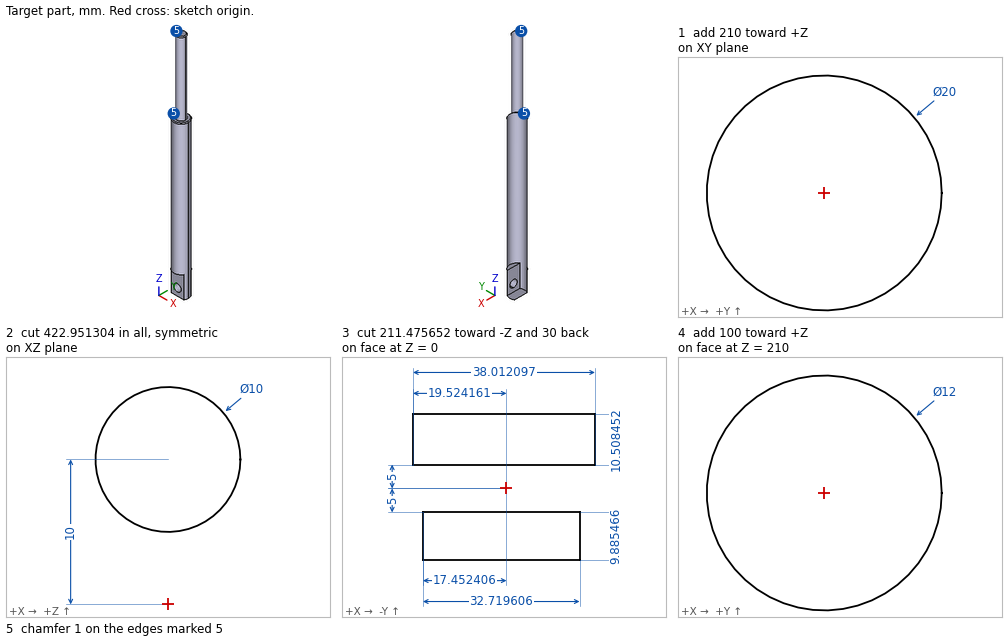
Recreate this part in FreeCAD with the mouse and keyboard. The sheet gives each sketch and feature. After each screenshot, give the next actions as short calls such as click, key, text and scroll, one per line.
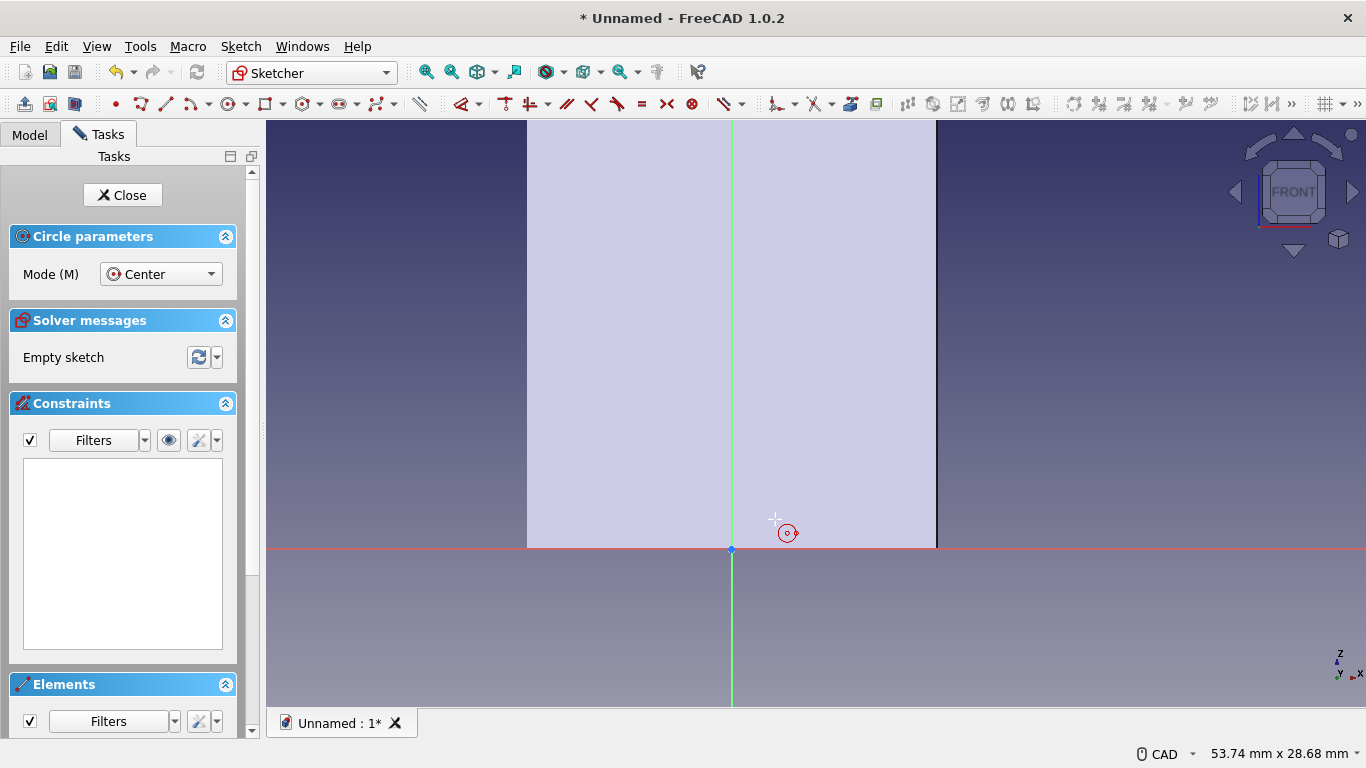
click(732, 344)
move(804, 272)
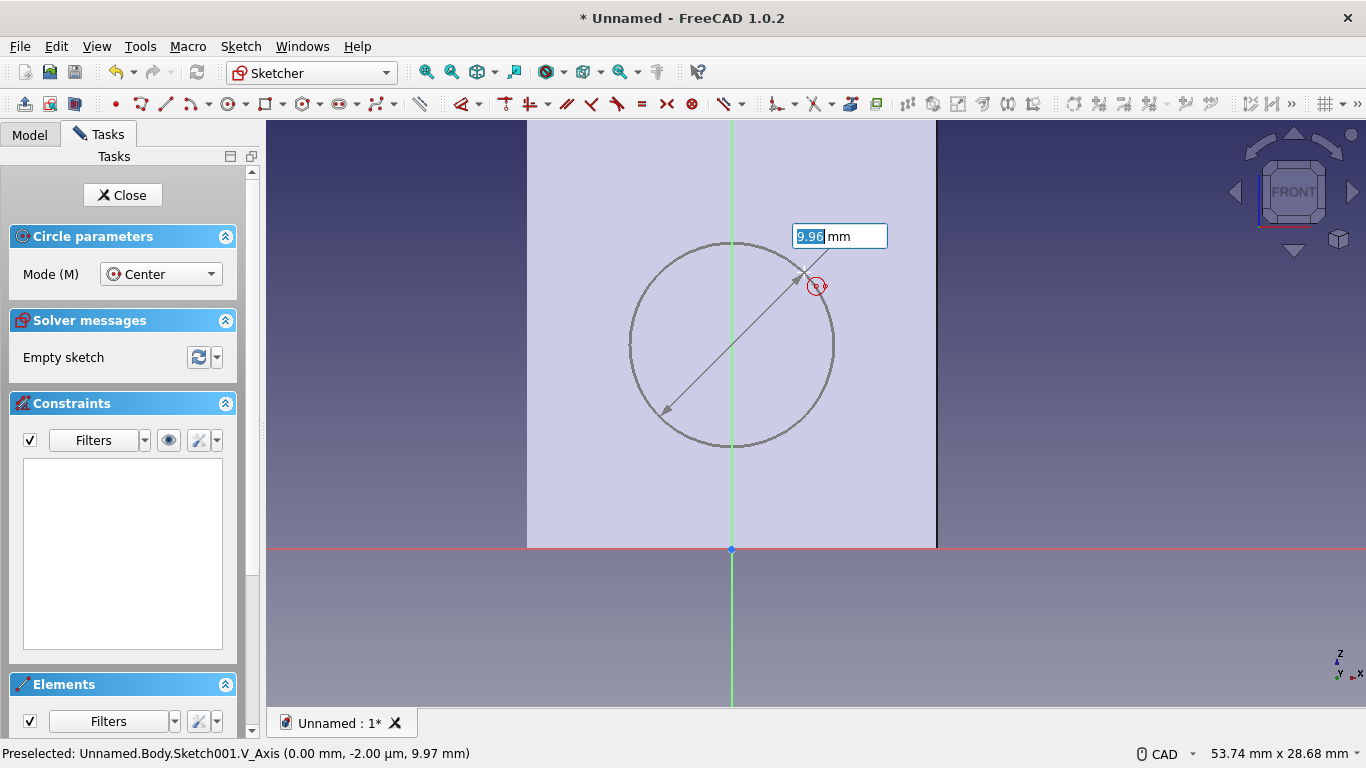
text(10)
key(Return)
key(Escape)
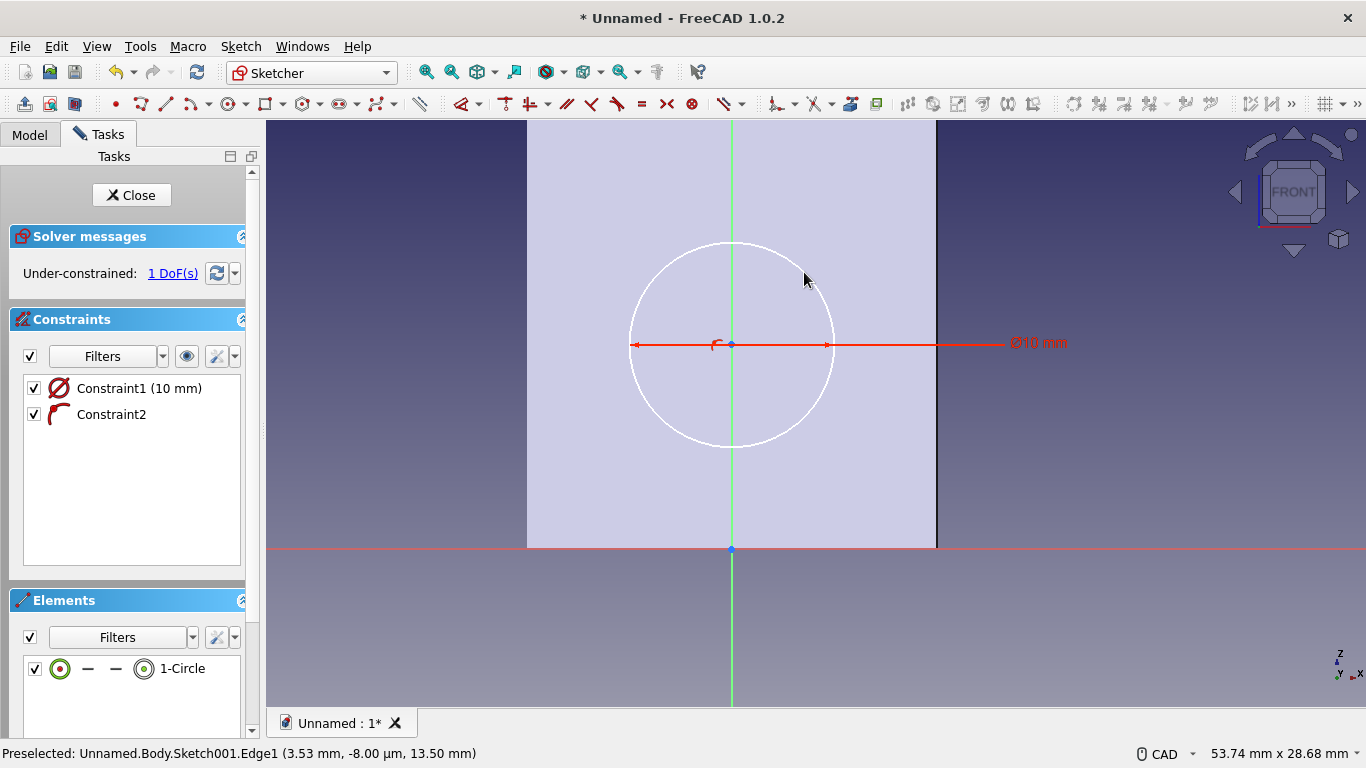
click(732, 345)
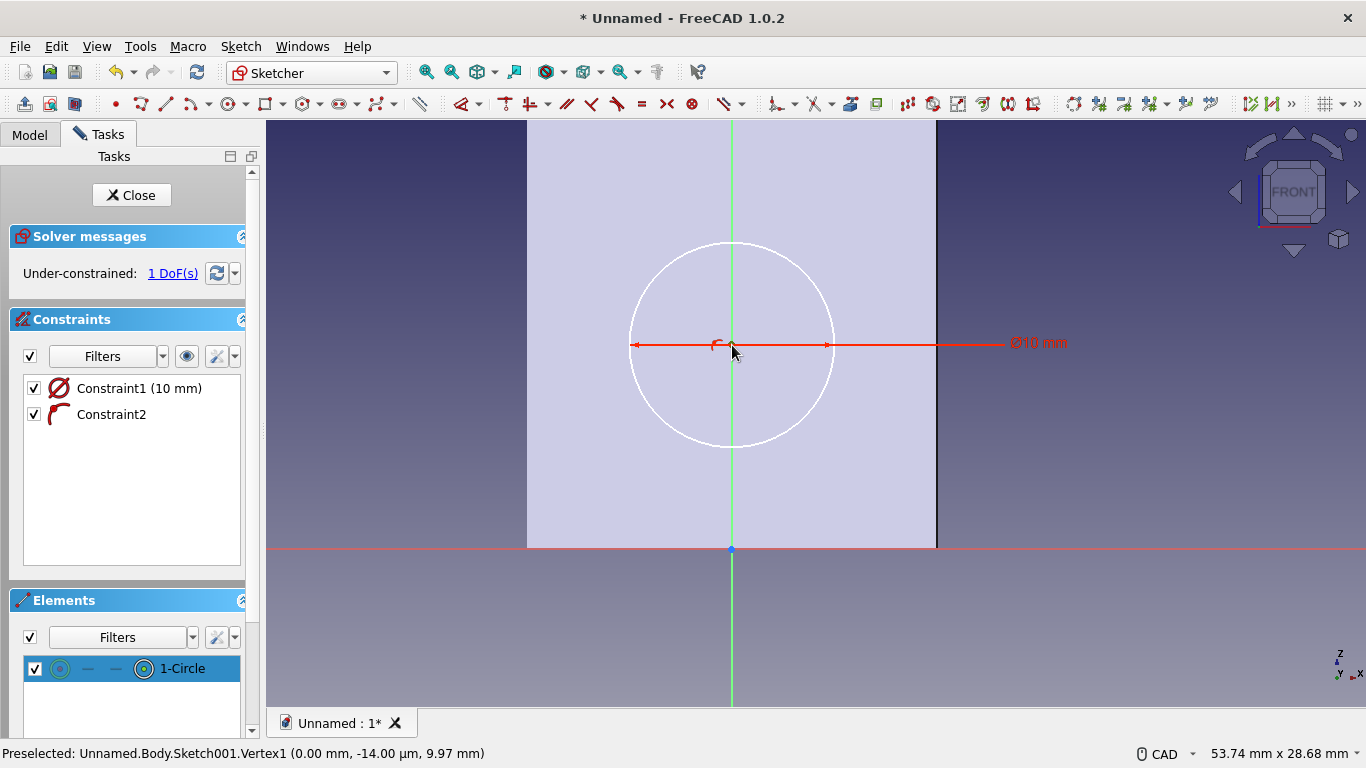
click(478, 104)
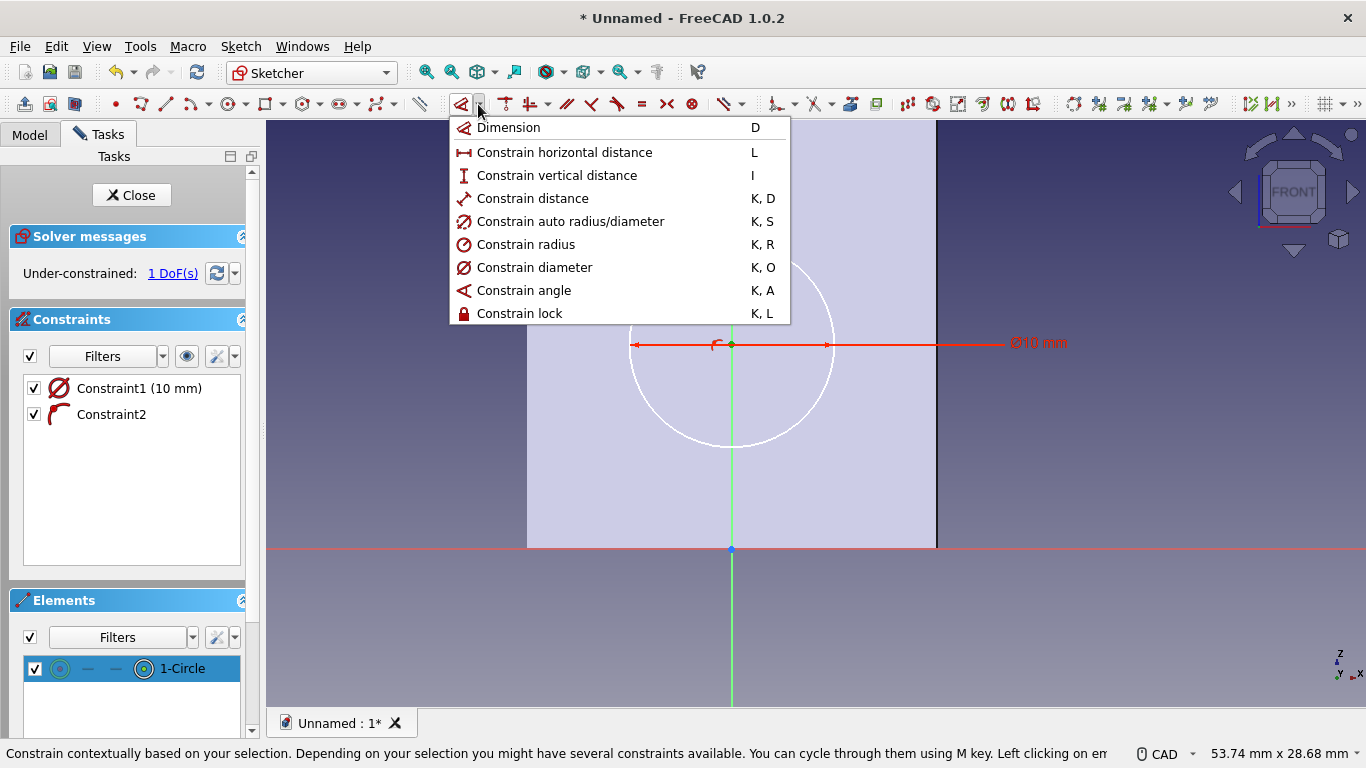
click(620, 176)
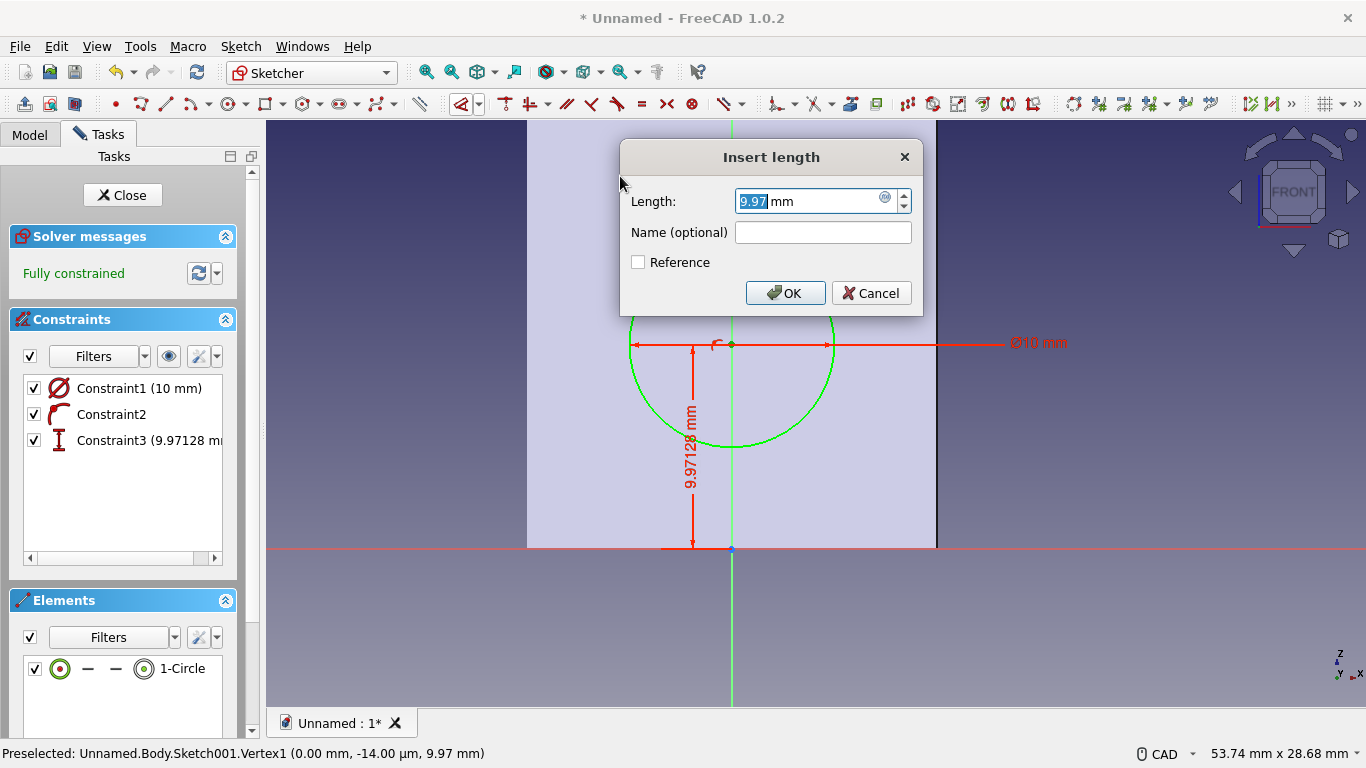
text(10)
key(Return)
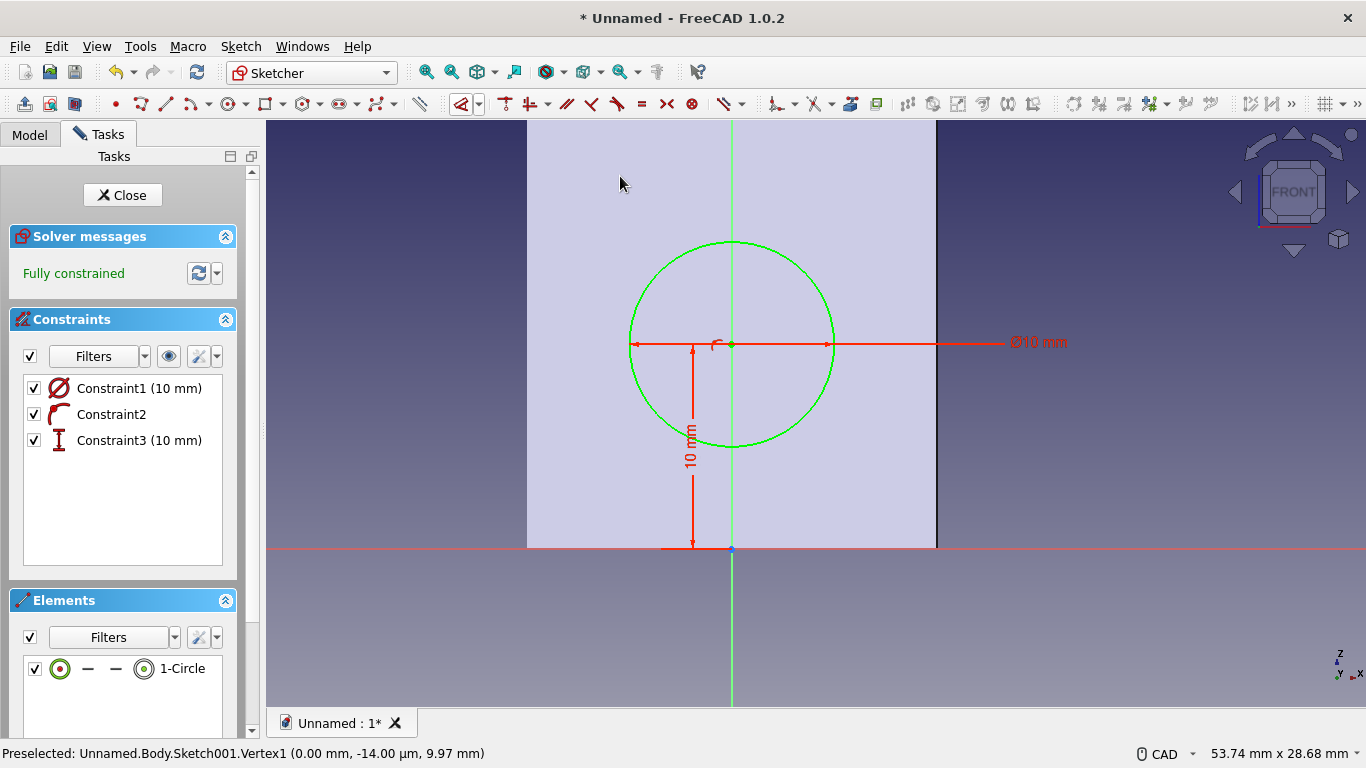
click(123, 195)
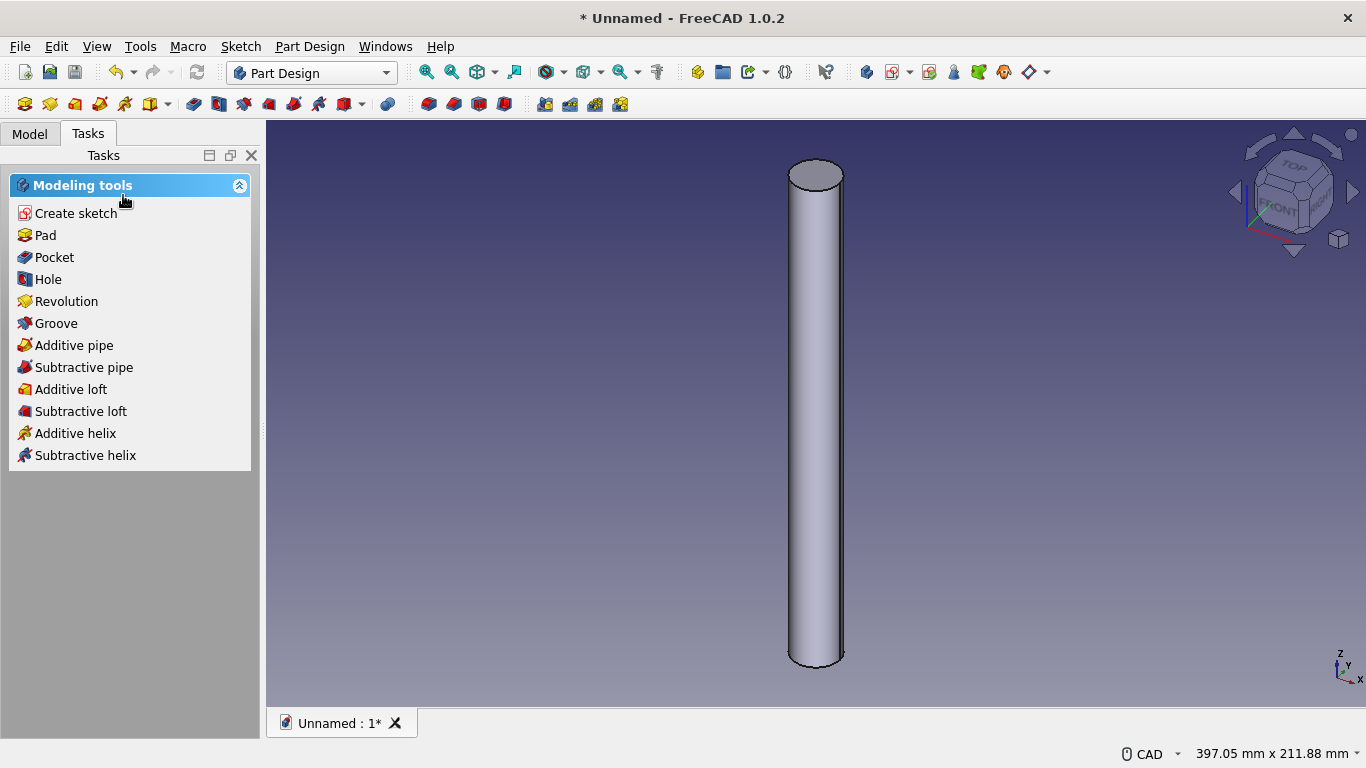
click(194, 104)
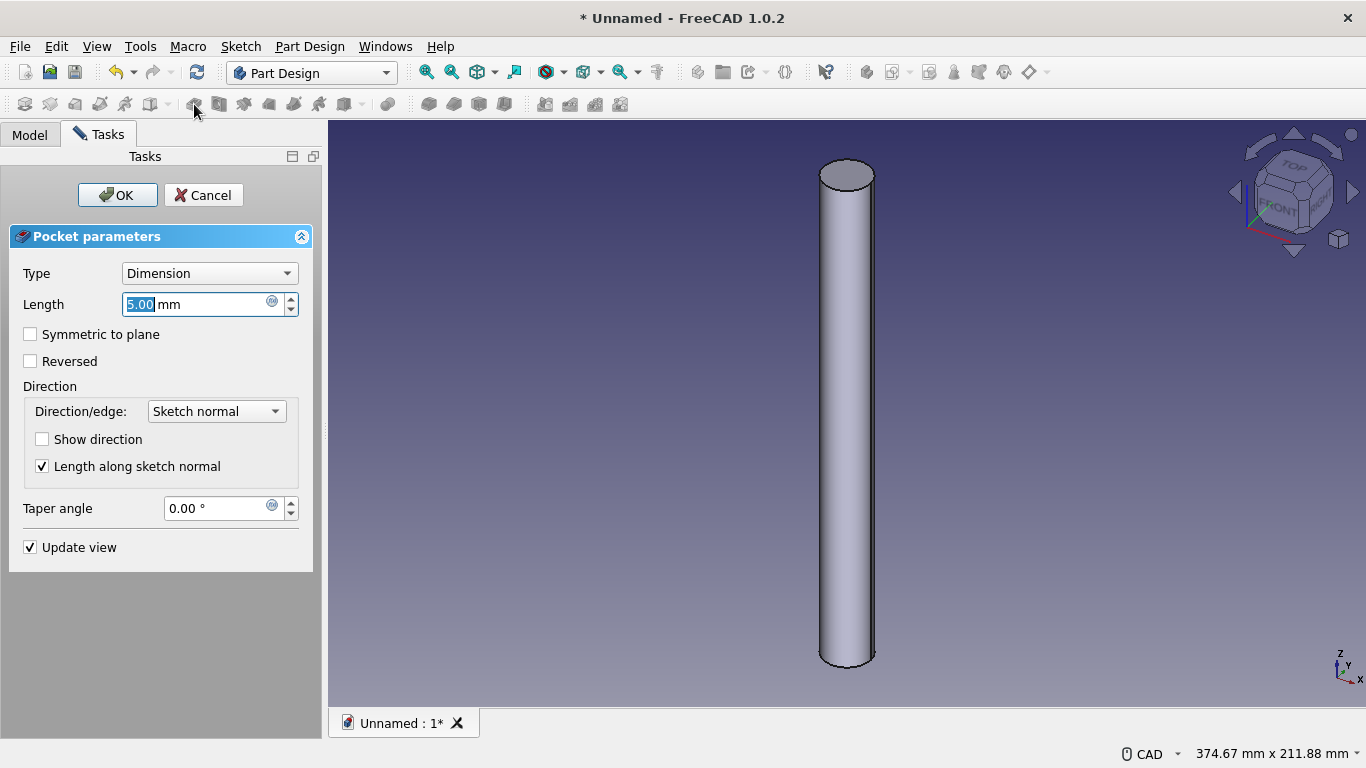
text(422.951304)
key(Tab)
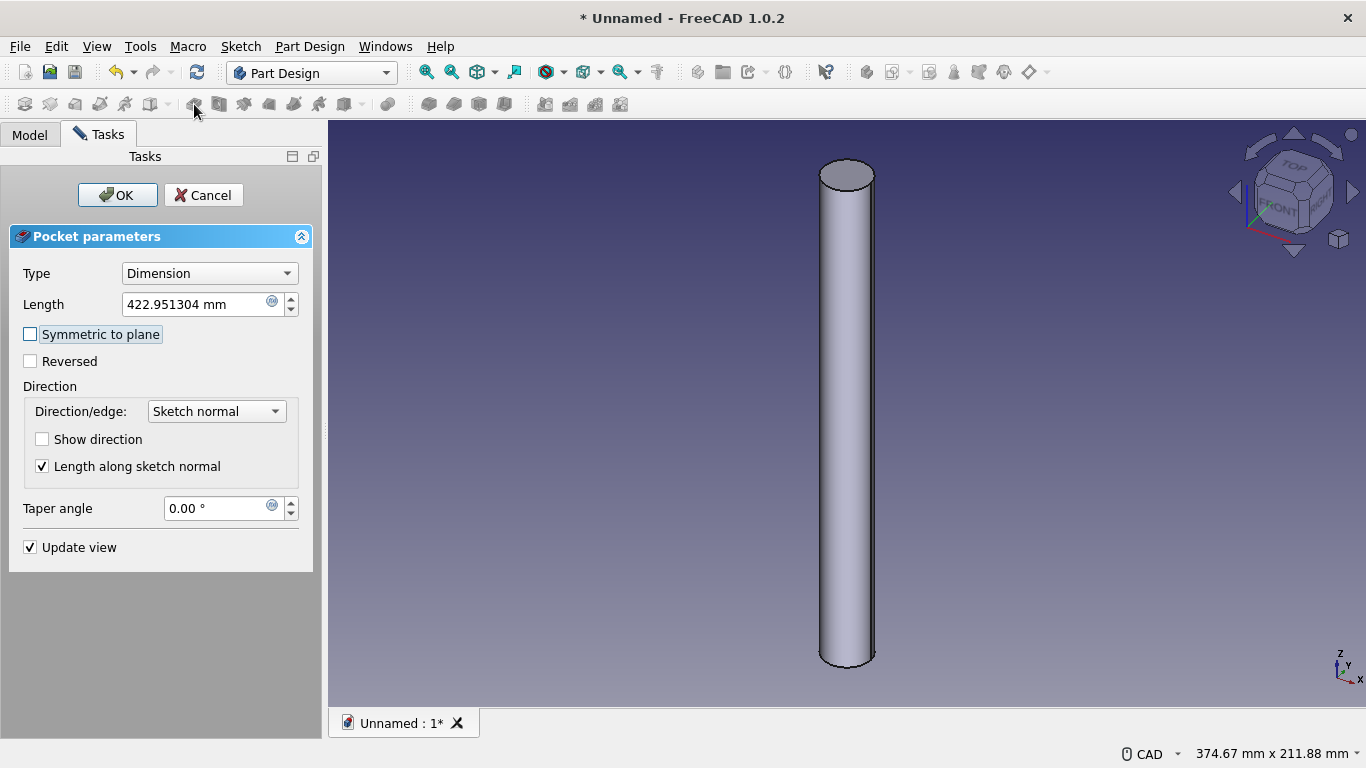
click(31, 334)